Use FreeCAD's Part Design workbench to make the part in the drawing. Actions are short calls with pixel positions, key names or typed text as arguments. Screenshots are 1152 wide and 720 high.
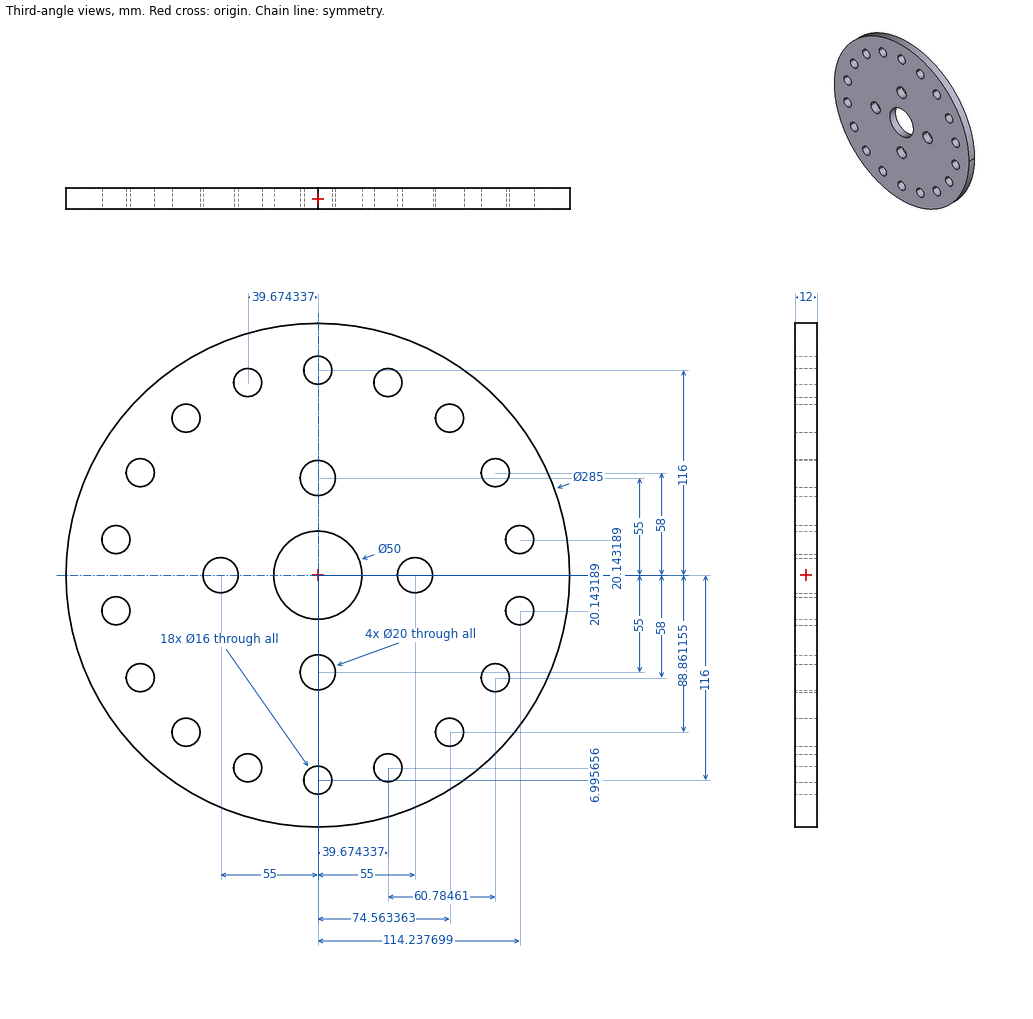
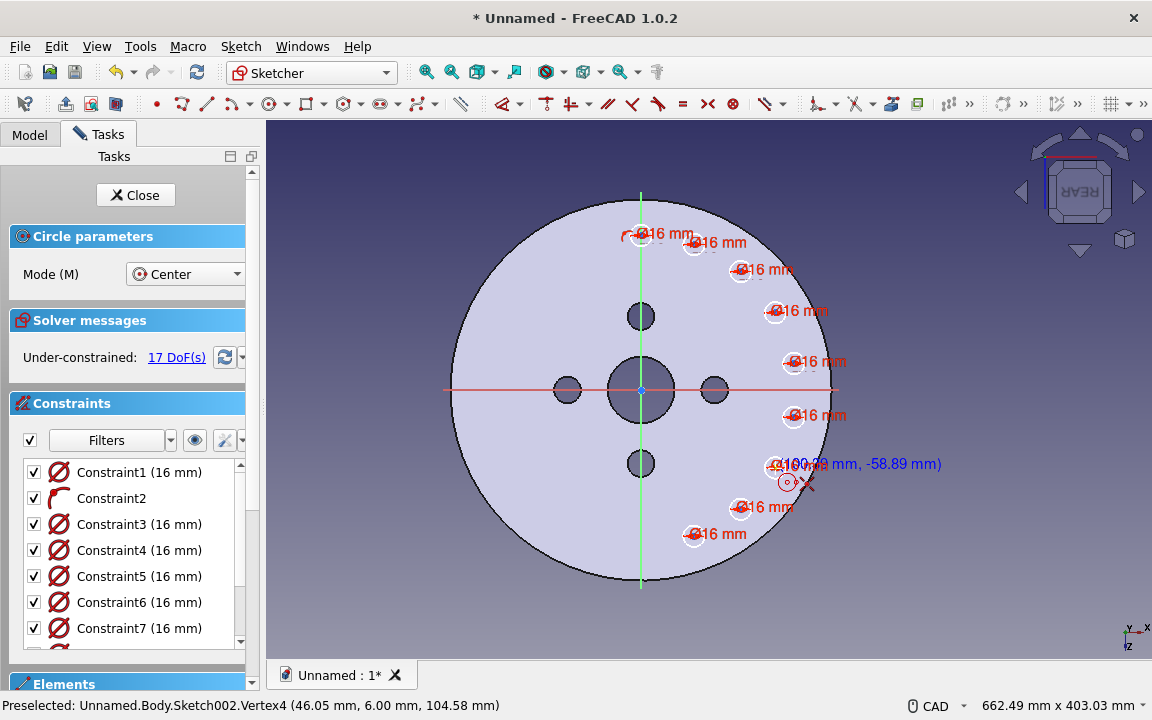
scroll(641, 545, up, 4)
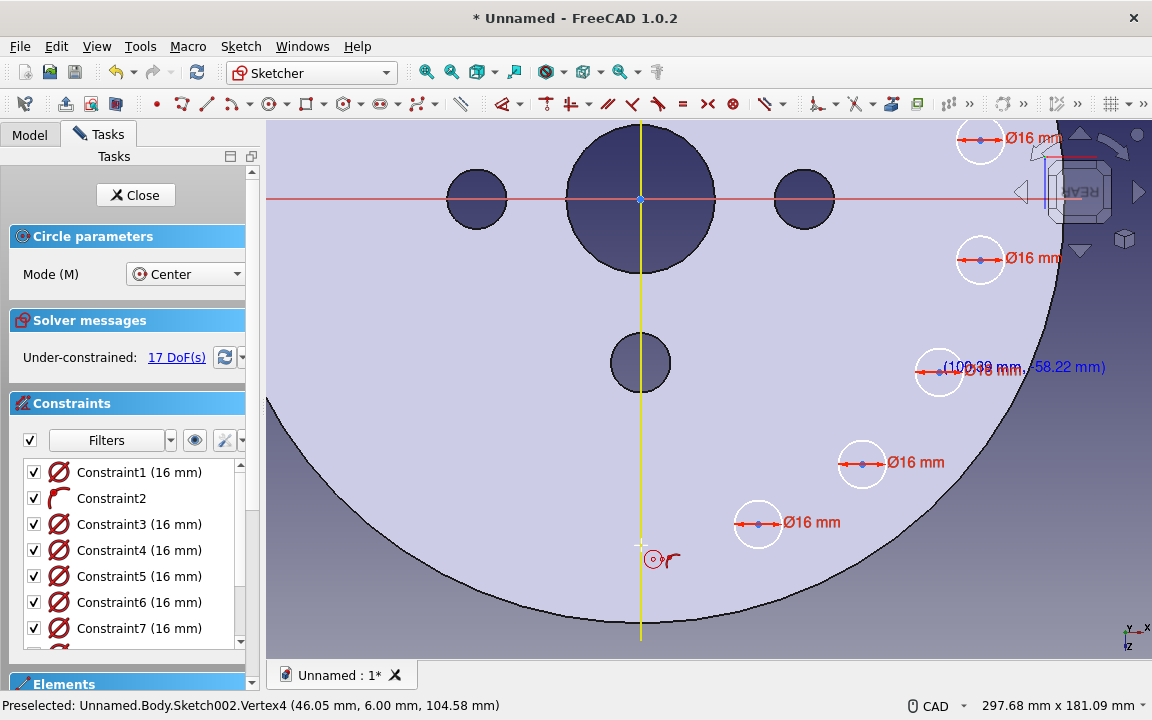
click(641, 544)
move(657, 528)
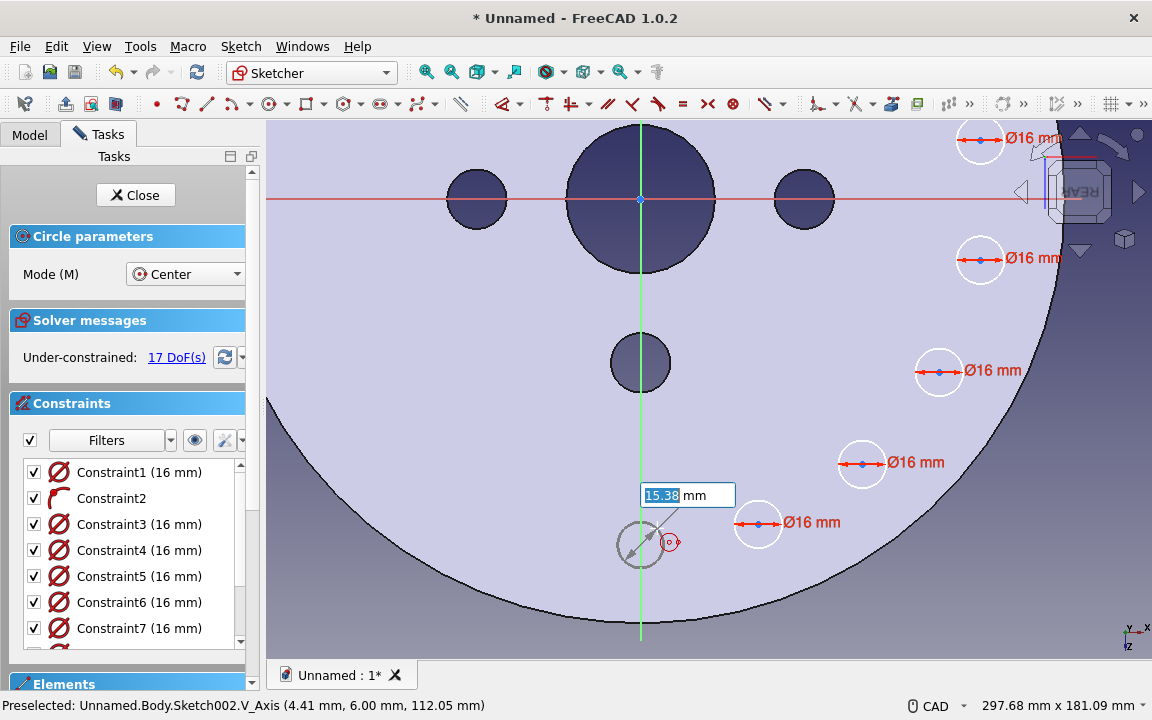
text(16)
key(Return)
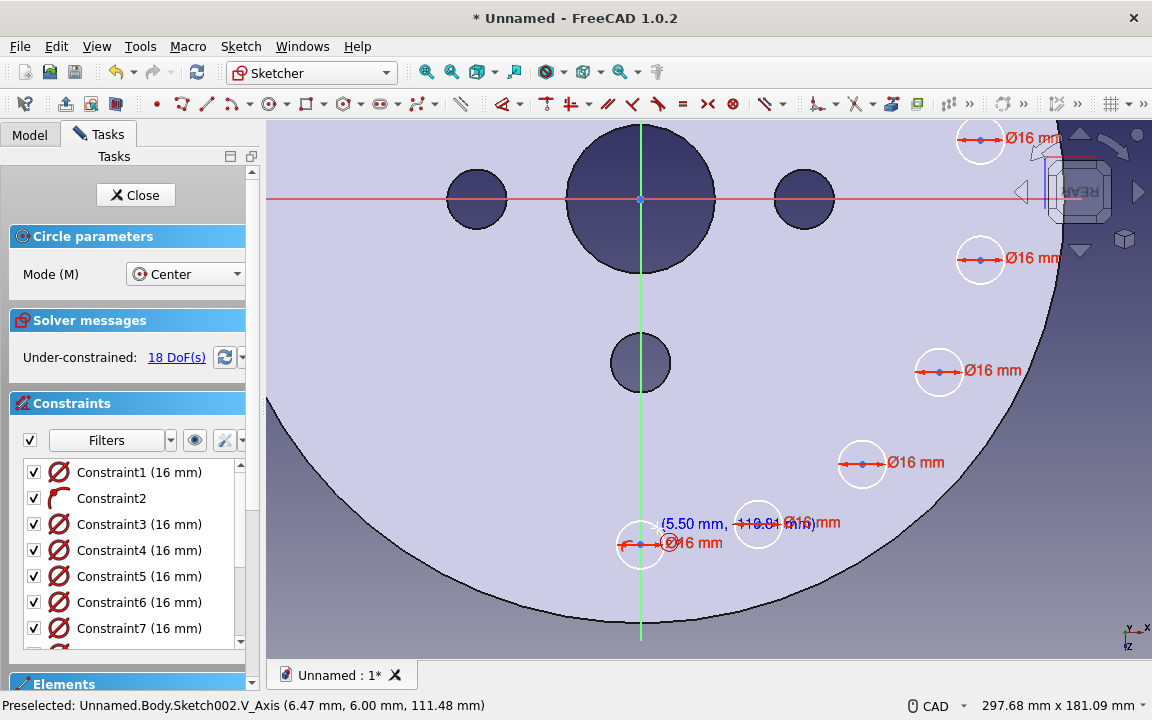
click(523, 524)
move(539, 507)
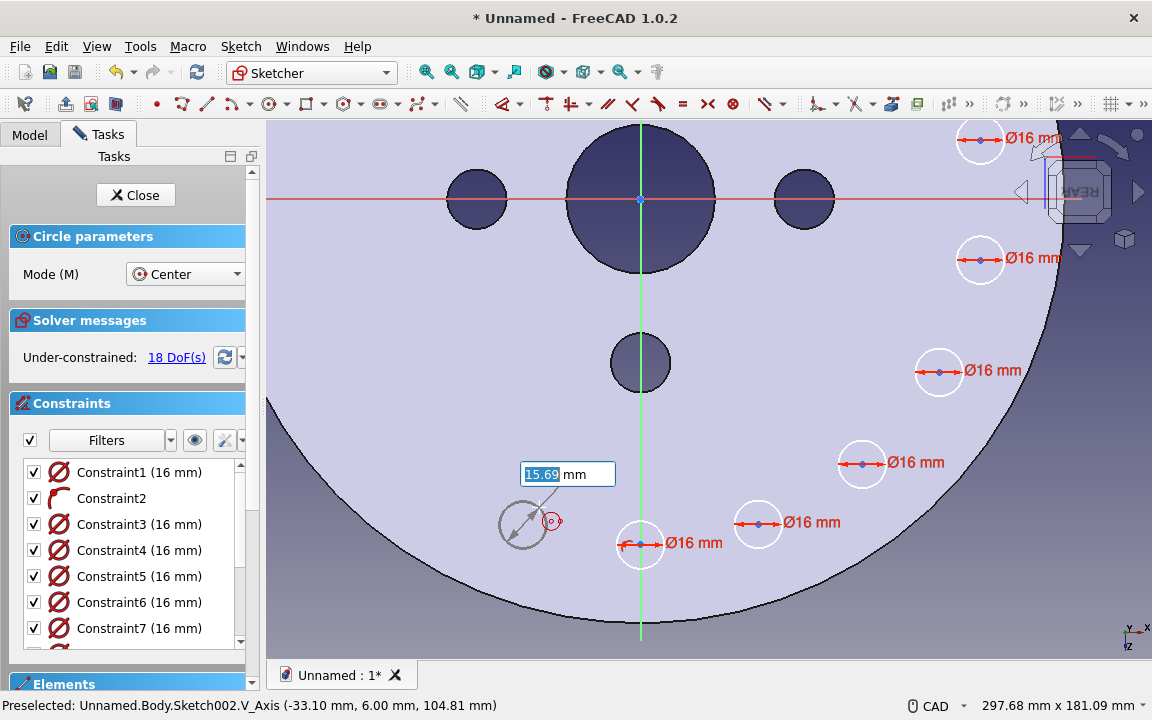
text(16)
key(Return)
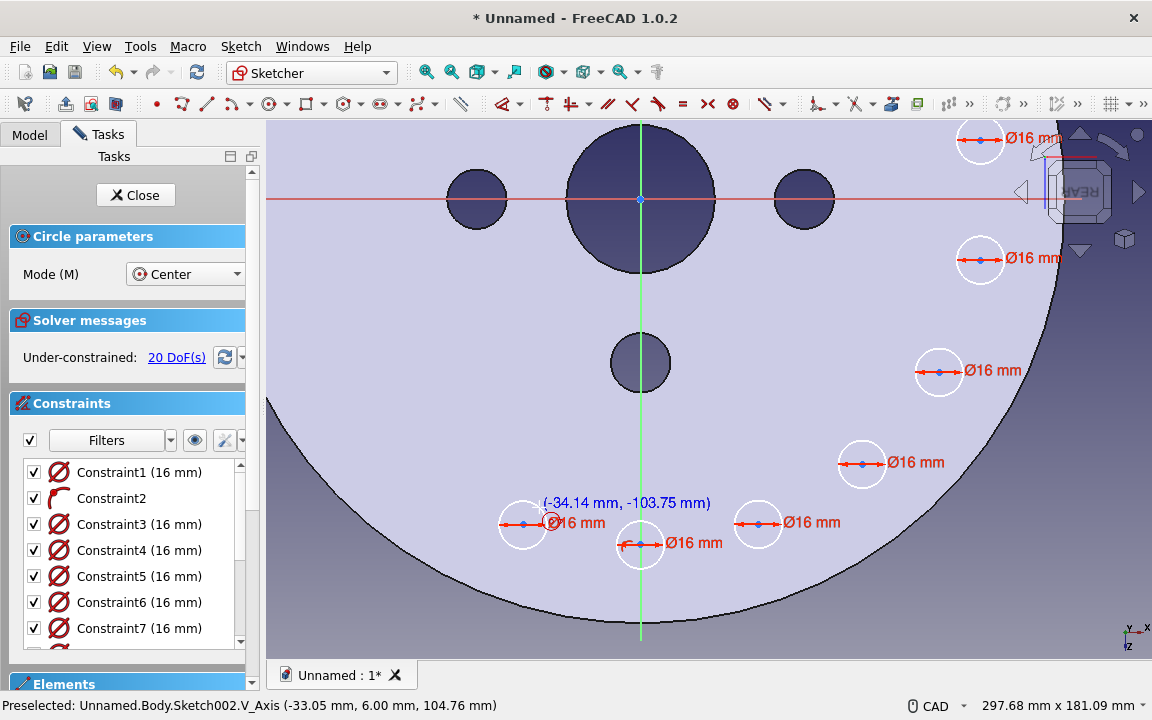
click(419, 464)
move(436, 447)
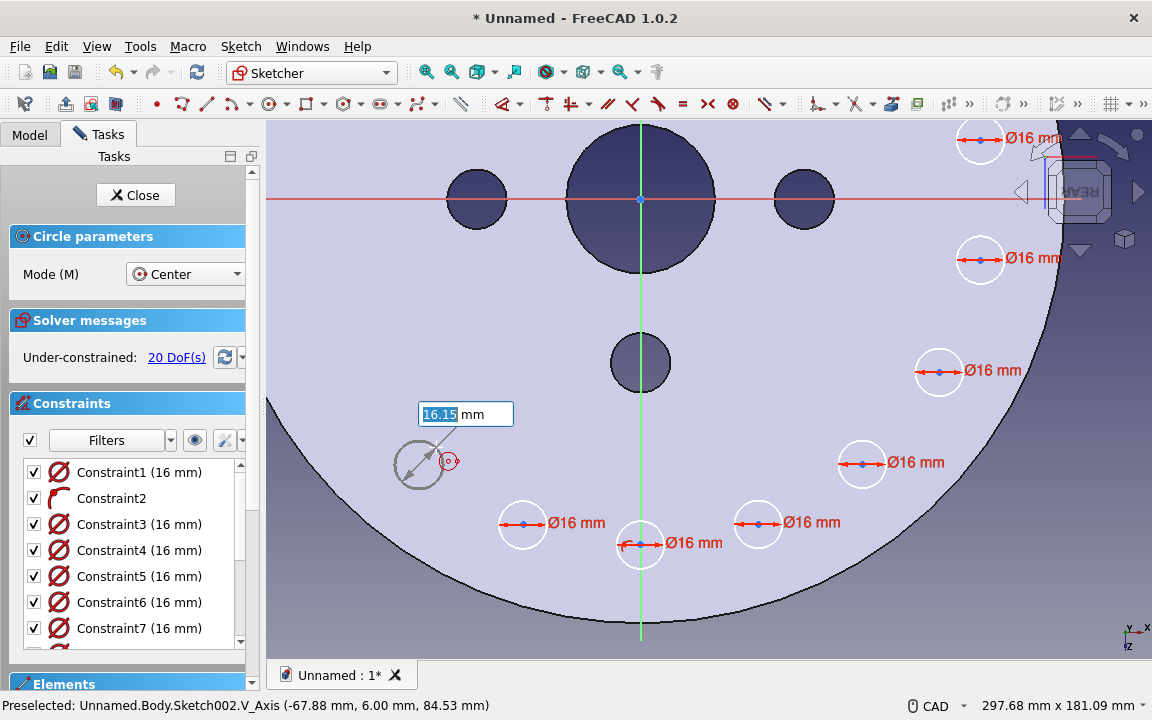
text(16)
key(Return)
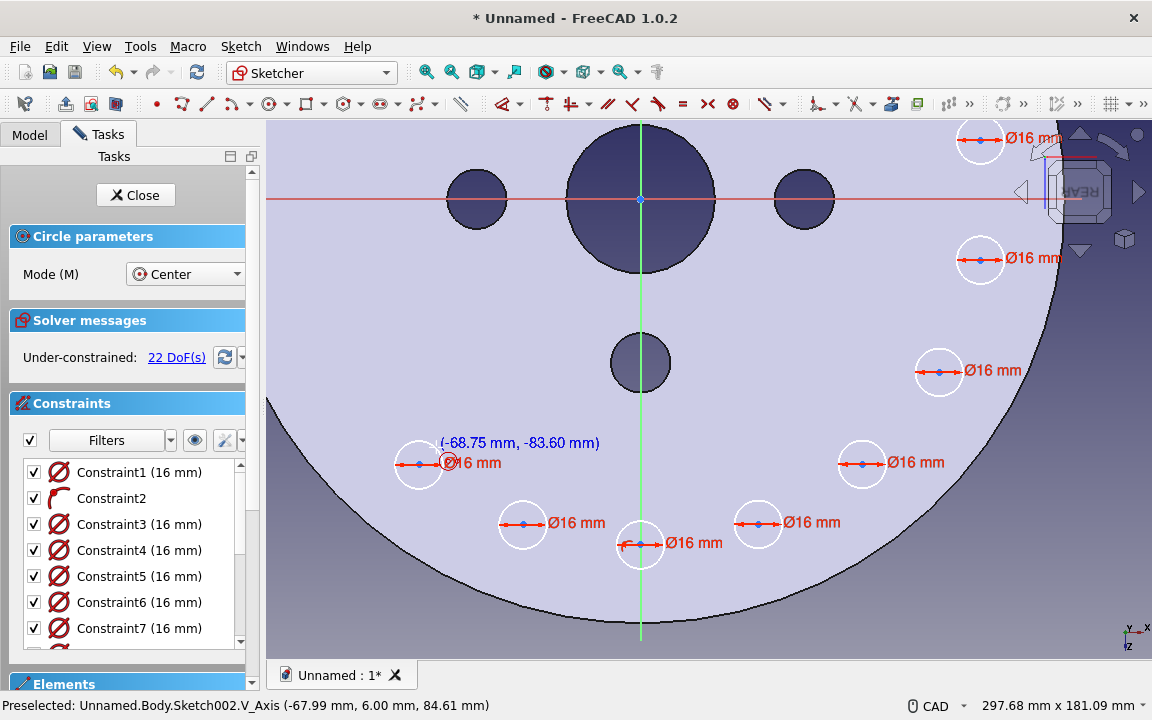
click(342, 372)
move(358, 355)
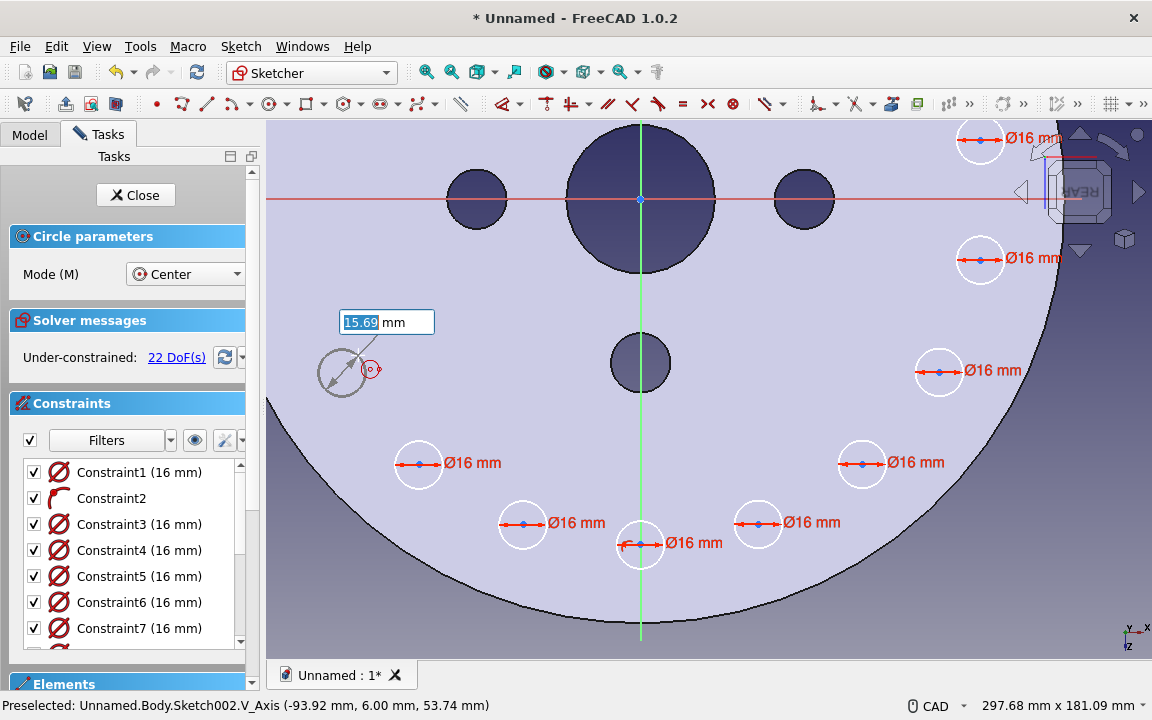
text(16)
key(Return)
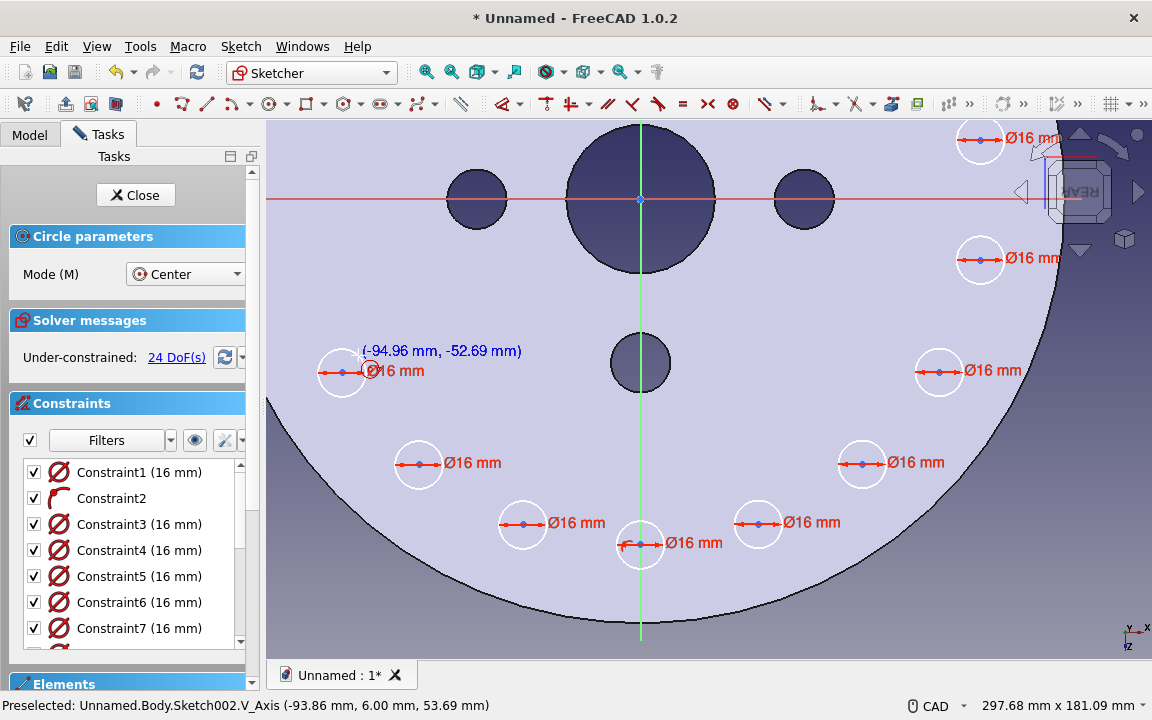
click(301, 259)
move(317, 242)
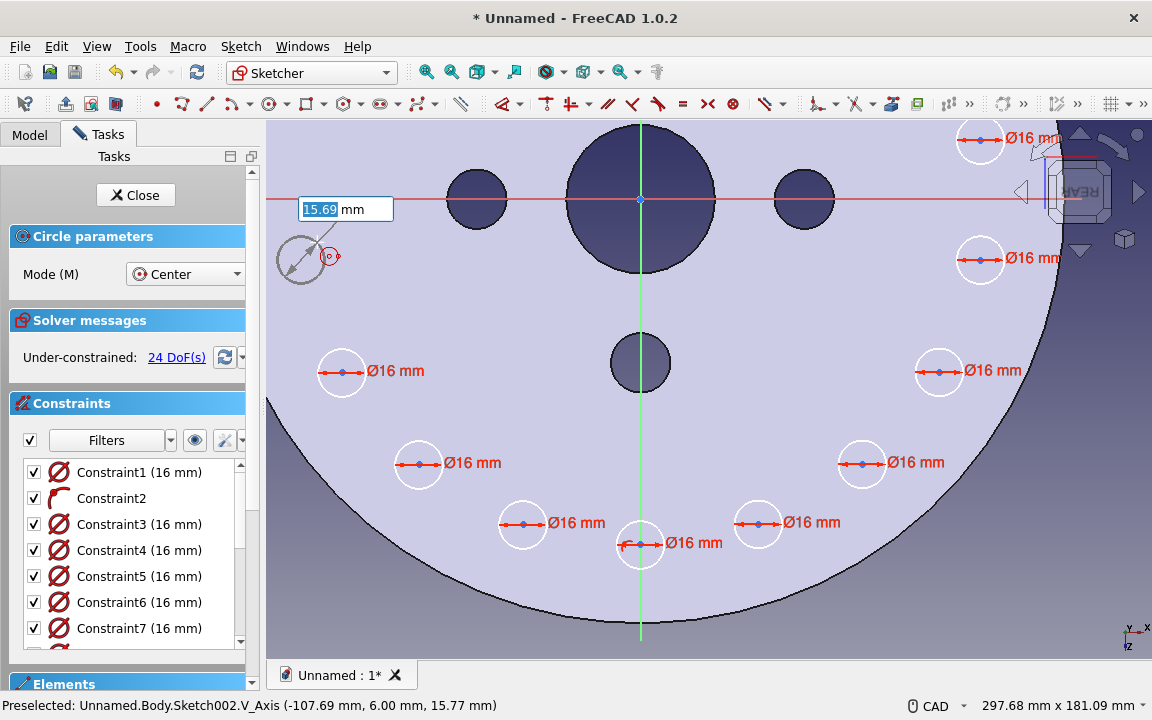
text(16)
key(Return)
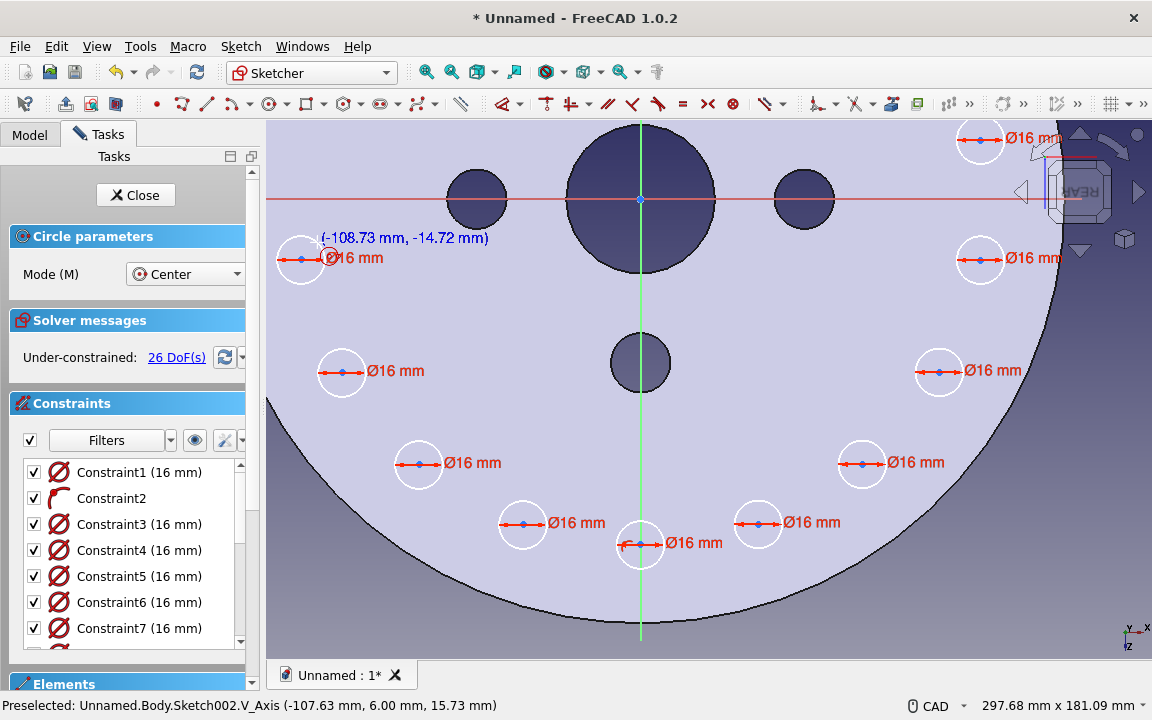
scroll(640, 545, down, 4)